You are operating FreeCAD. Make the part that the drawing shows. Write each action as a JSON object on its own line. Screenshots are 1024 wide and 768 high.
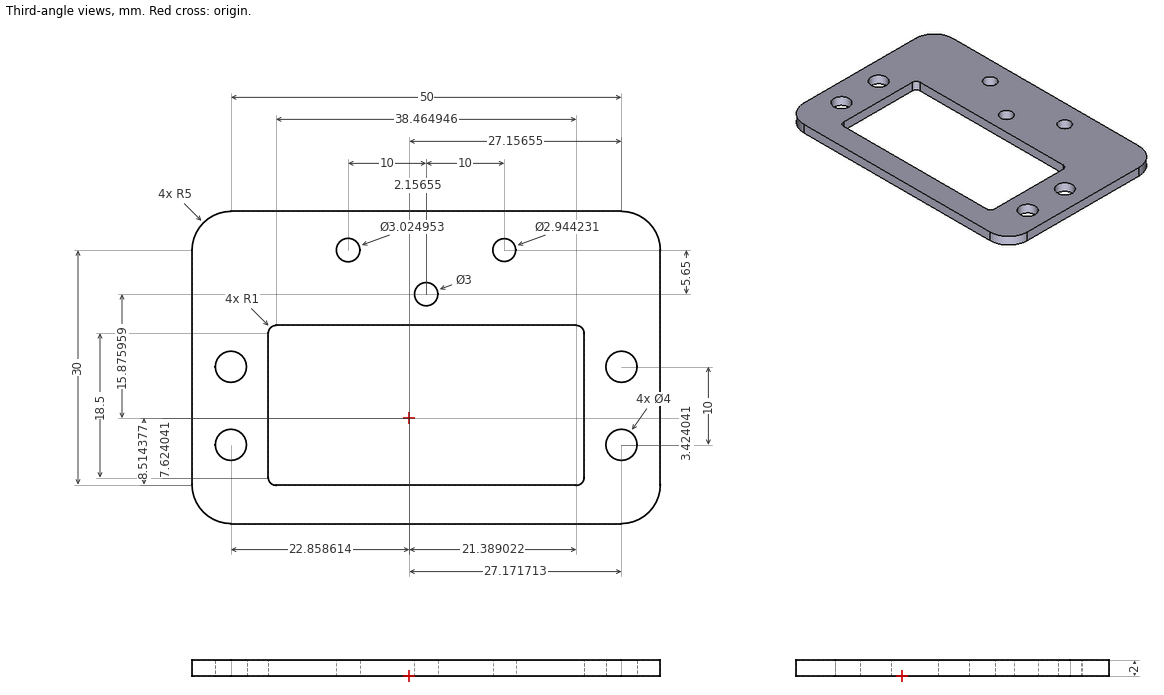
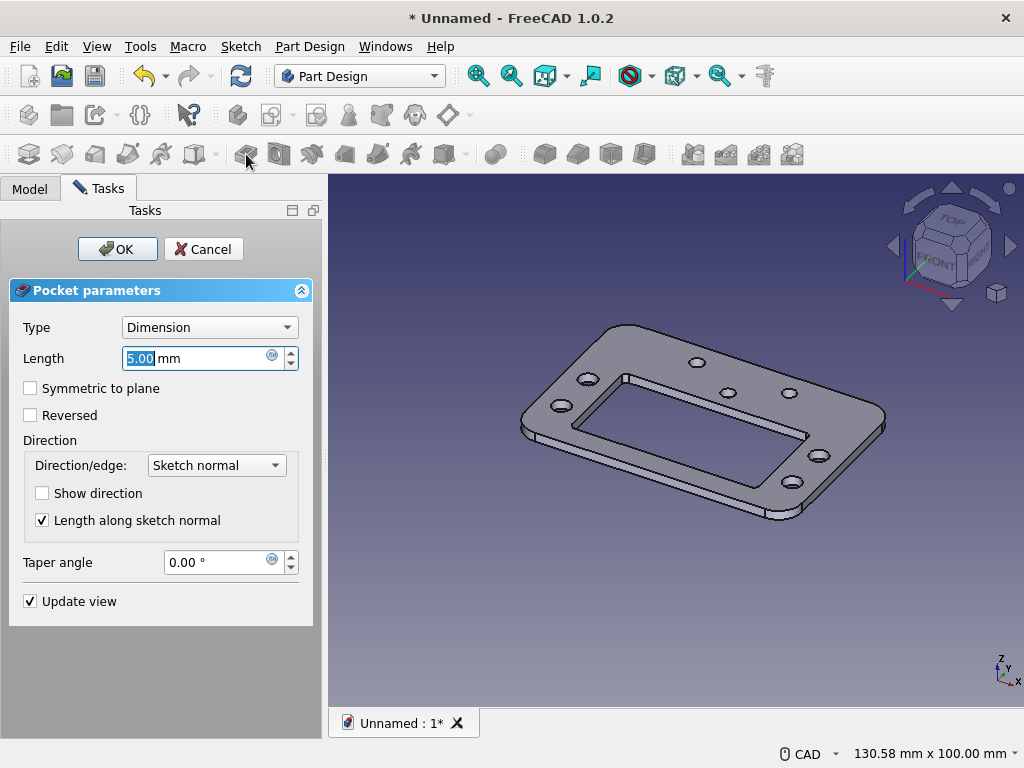
{"action": "left_click", "coordinate": [210, 328]}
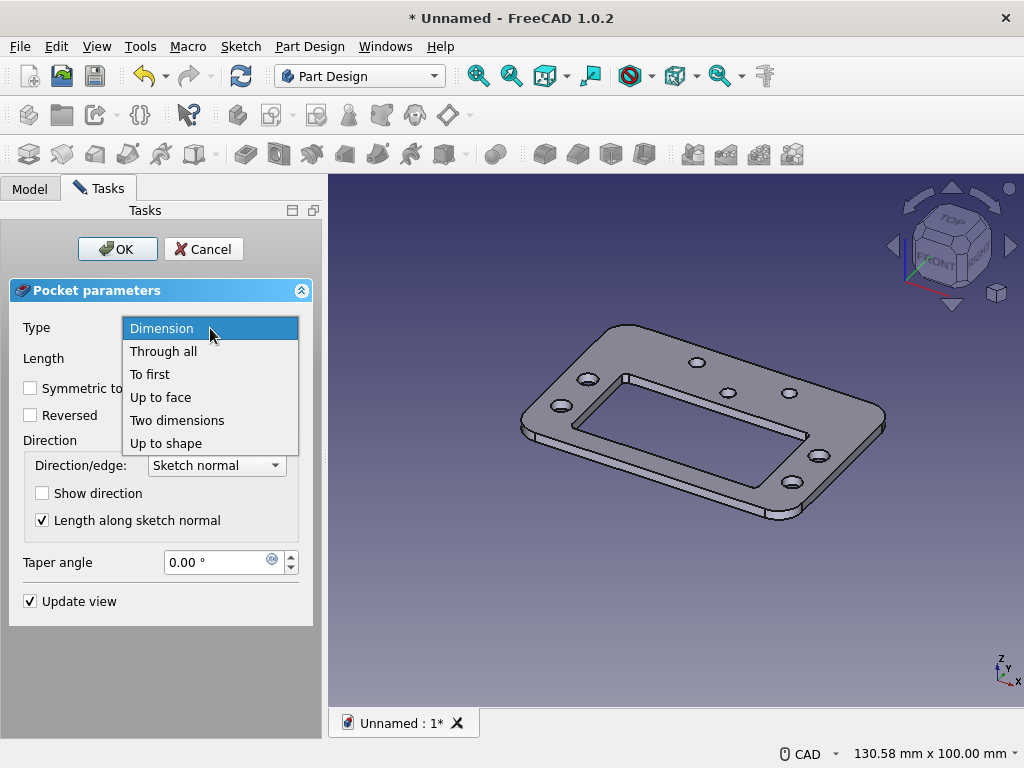
{"action": "left_click", "coordinate": [208, 352]}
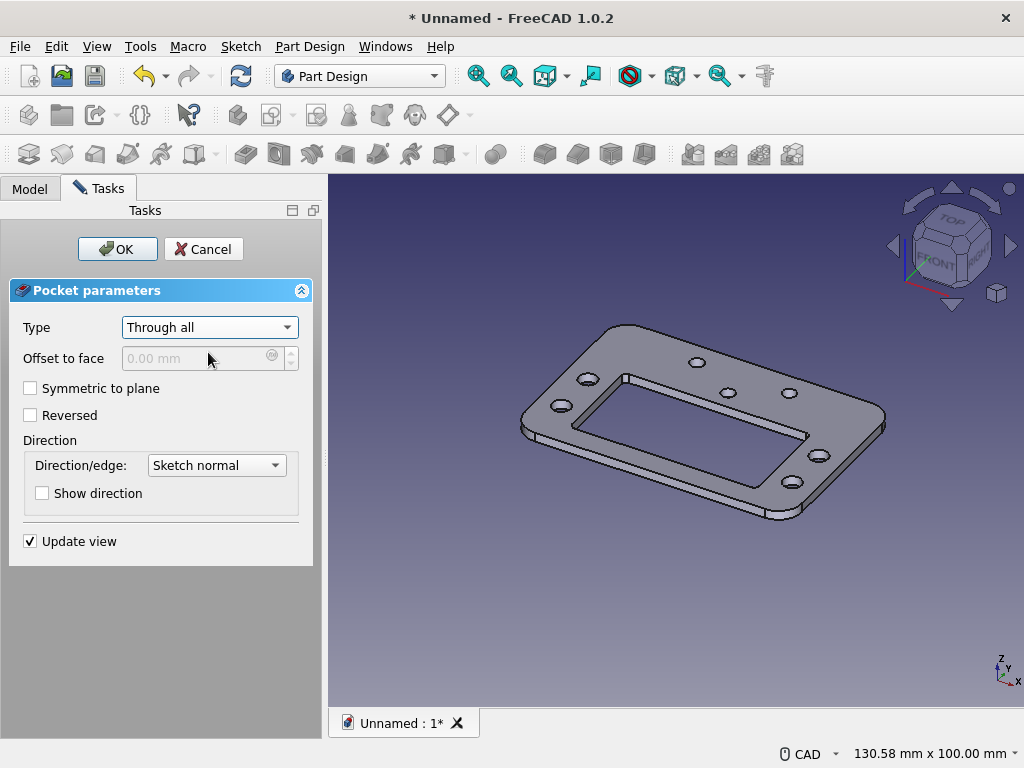
{"action": "left_click", "coordinate": [118, 249]}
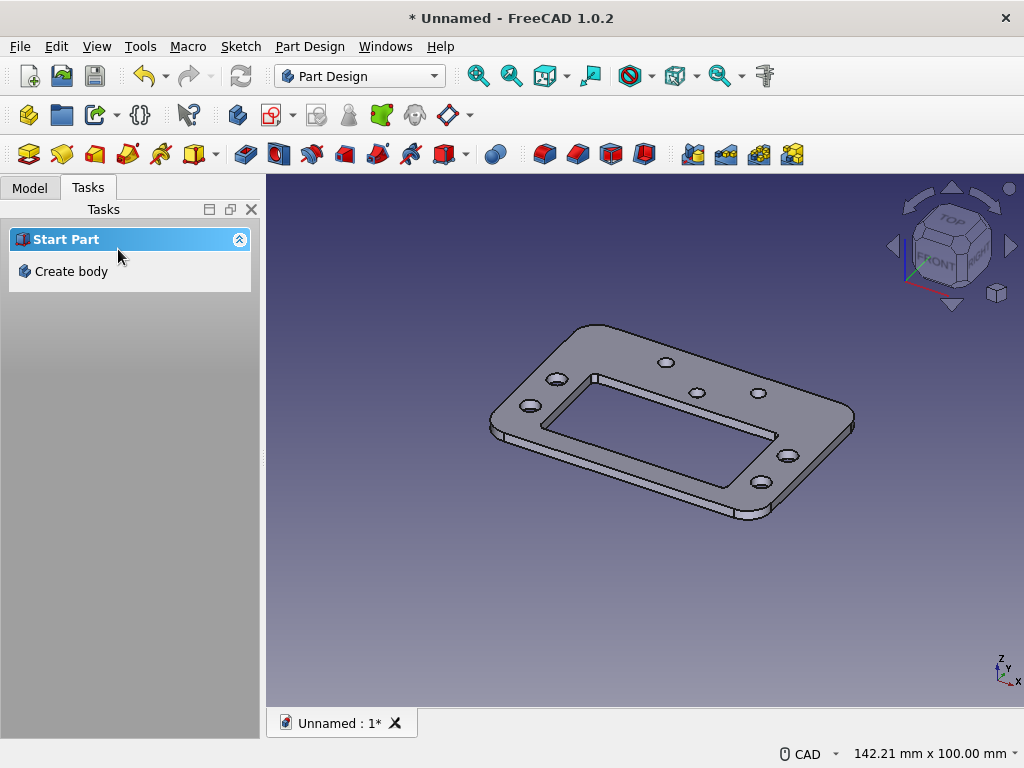
{"action": "key", "text": "0"}